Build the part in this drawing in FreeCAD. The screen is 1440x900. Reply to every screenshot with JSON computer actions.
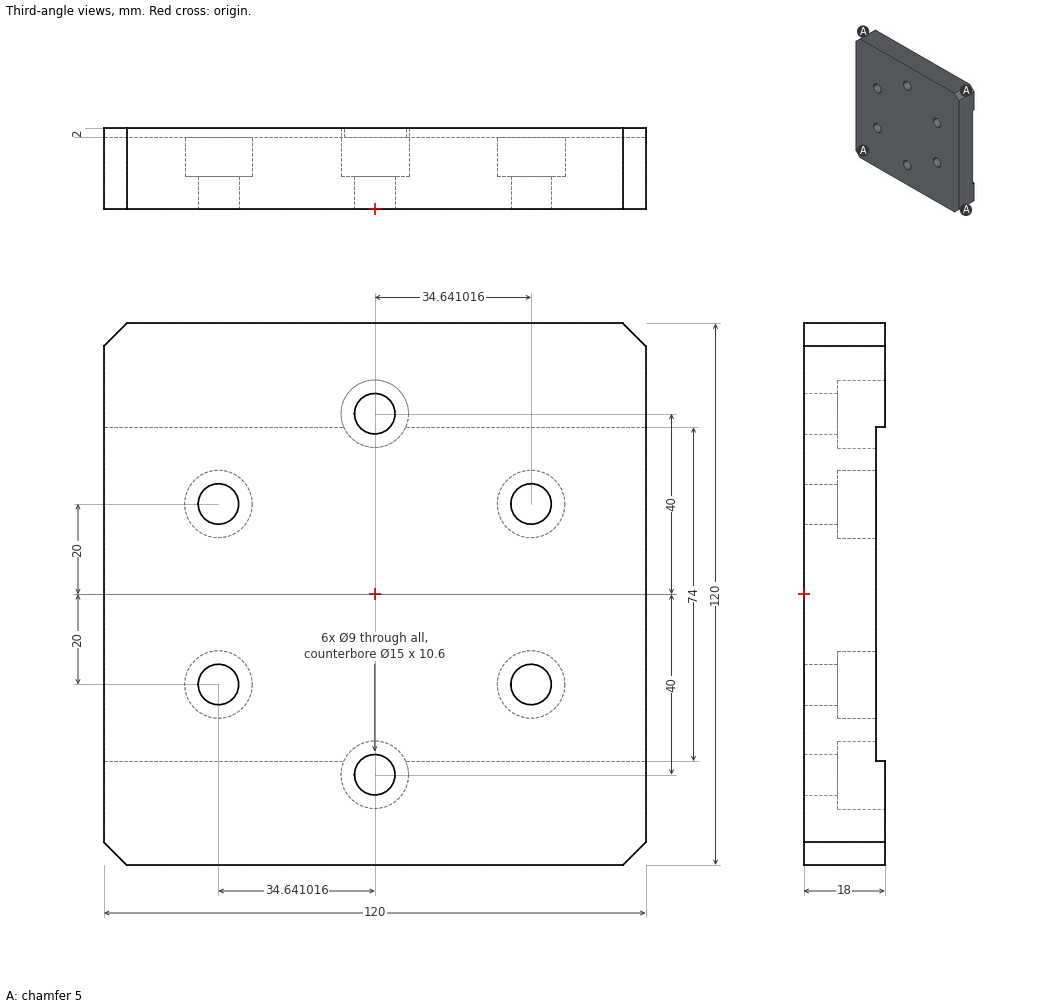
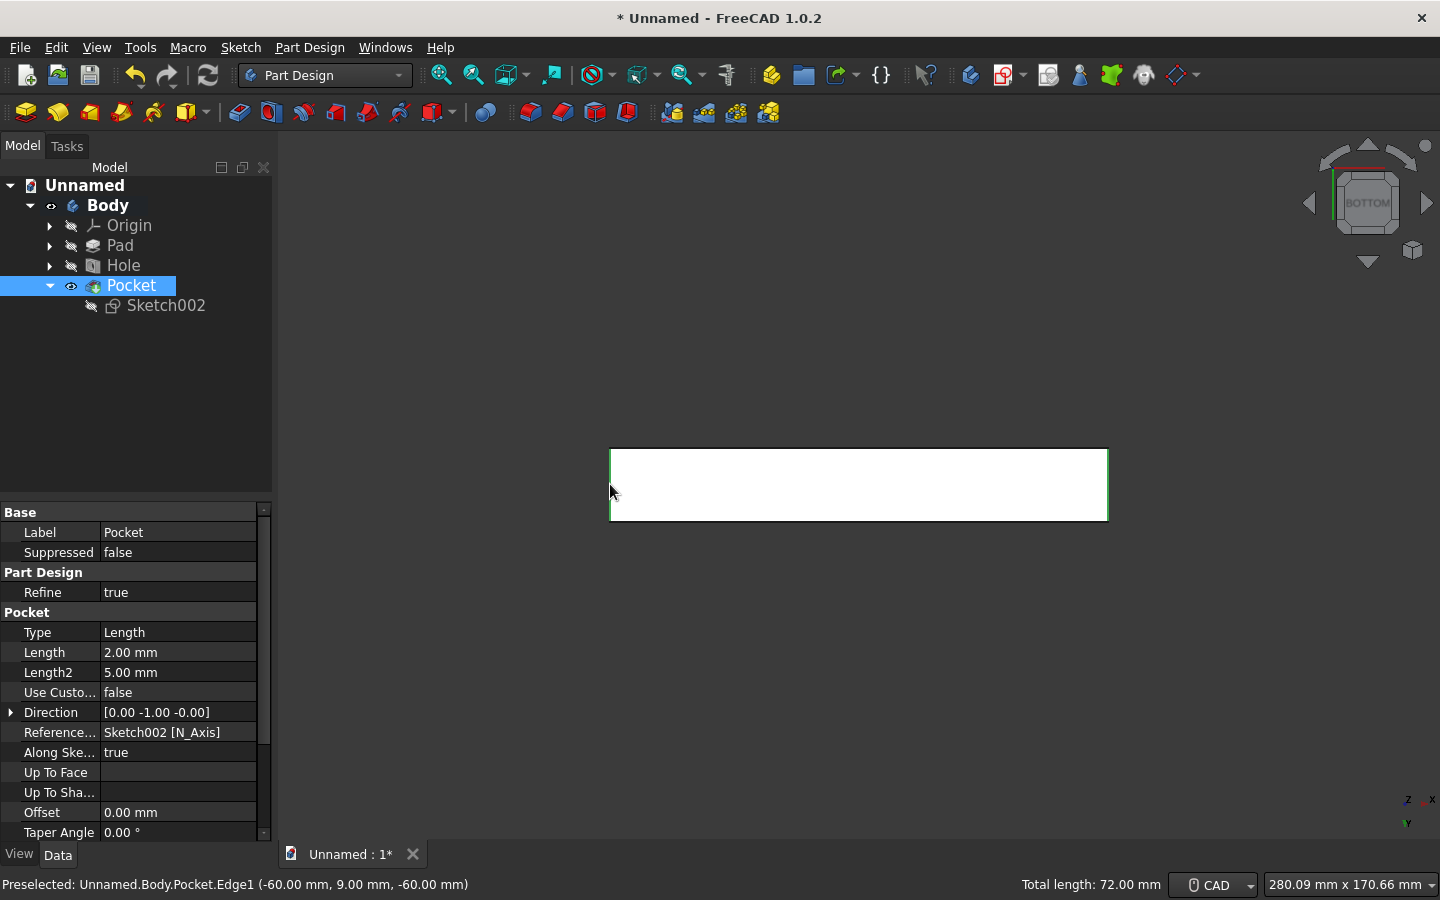
{"action": "left_click", "coordinate": [564, 112]}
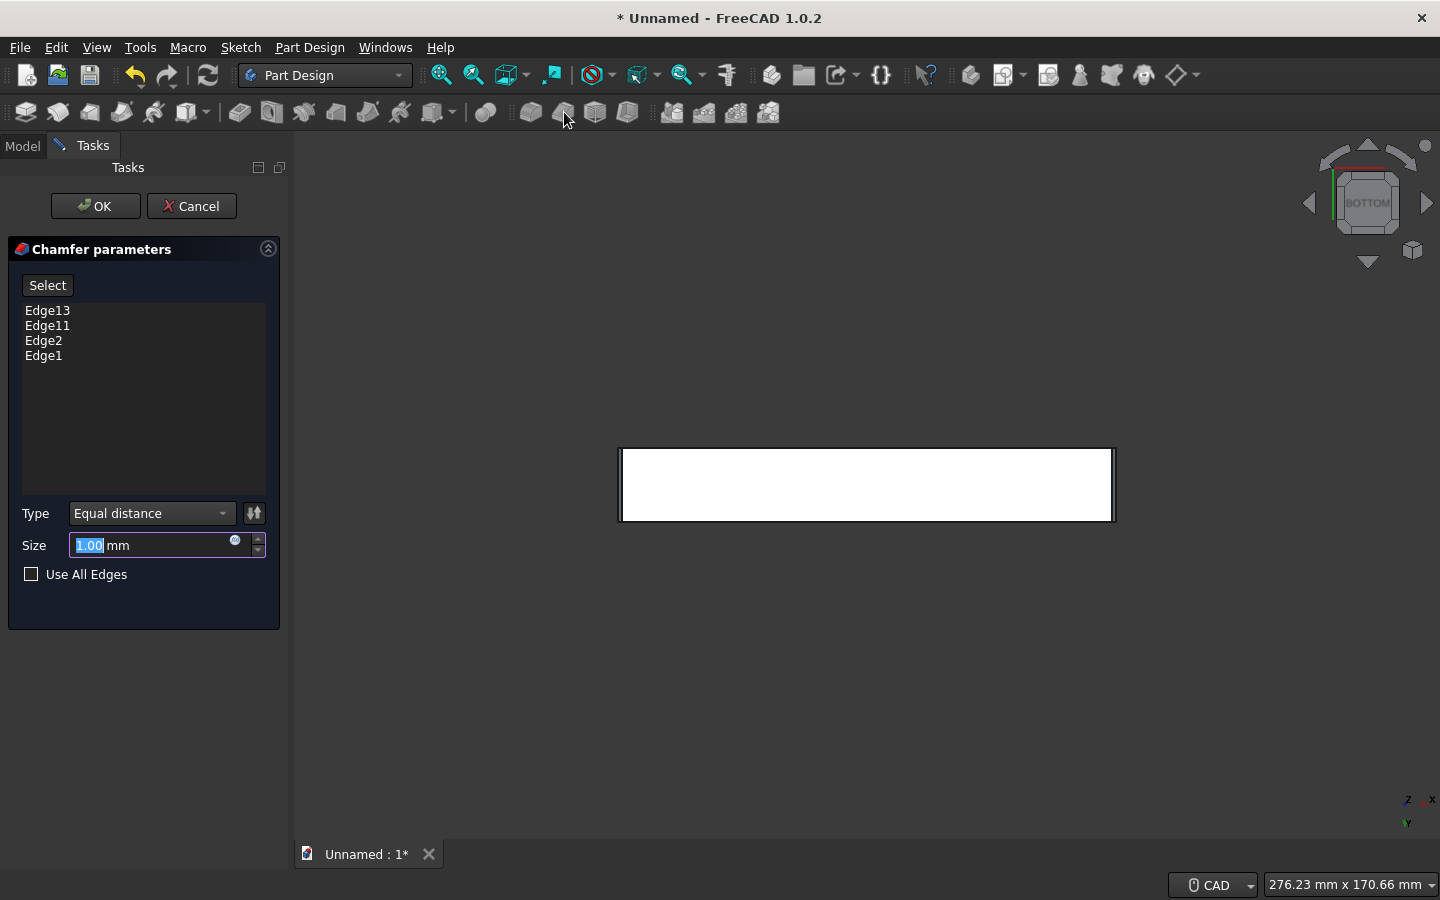
{"action": "type", "text": "5"}
{"action": "key", "text": "Tab"}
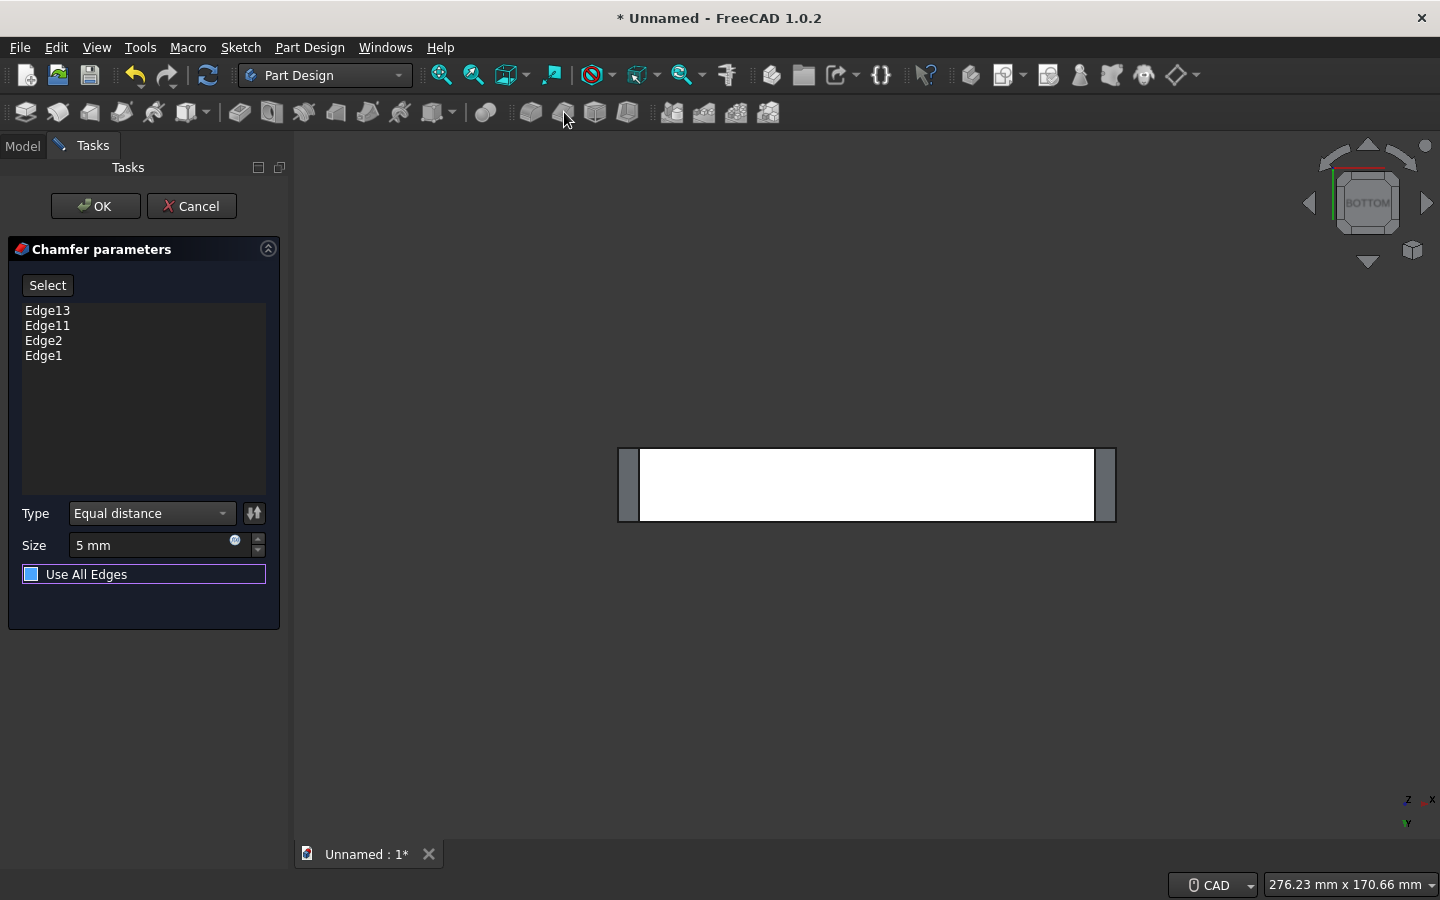
{"action": "left_click", "coordinate": [96, 206]}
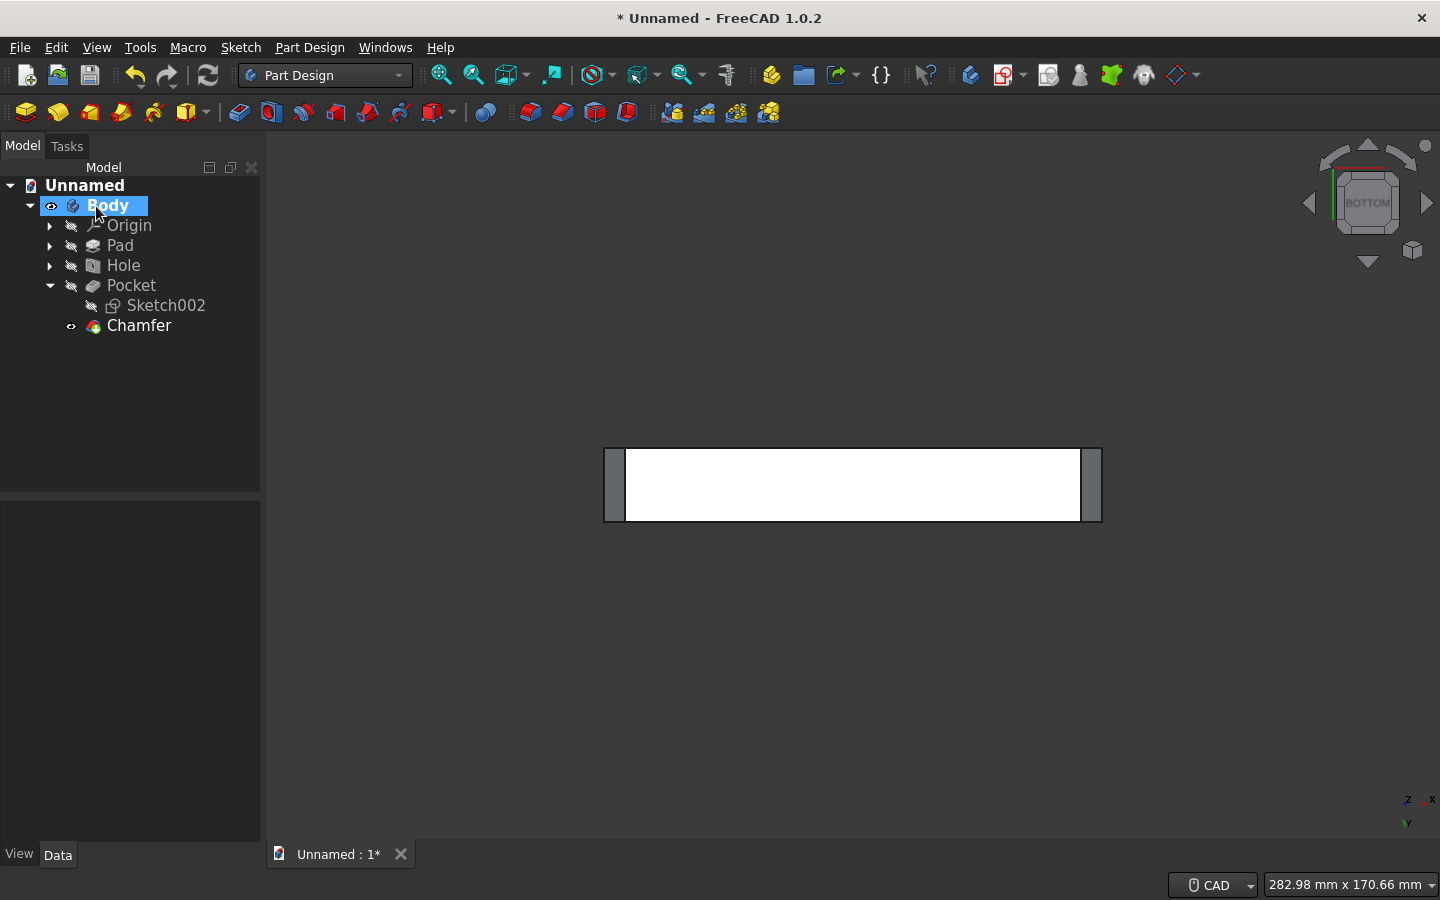
{"action": "key", "text": "0"}